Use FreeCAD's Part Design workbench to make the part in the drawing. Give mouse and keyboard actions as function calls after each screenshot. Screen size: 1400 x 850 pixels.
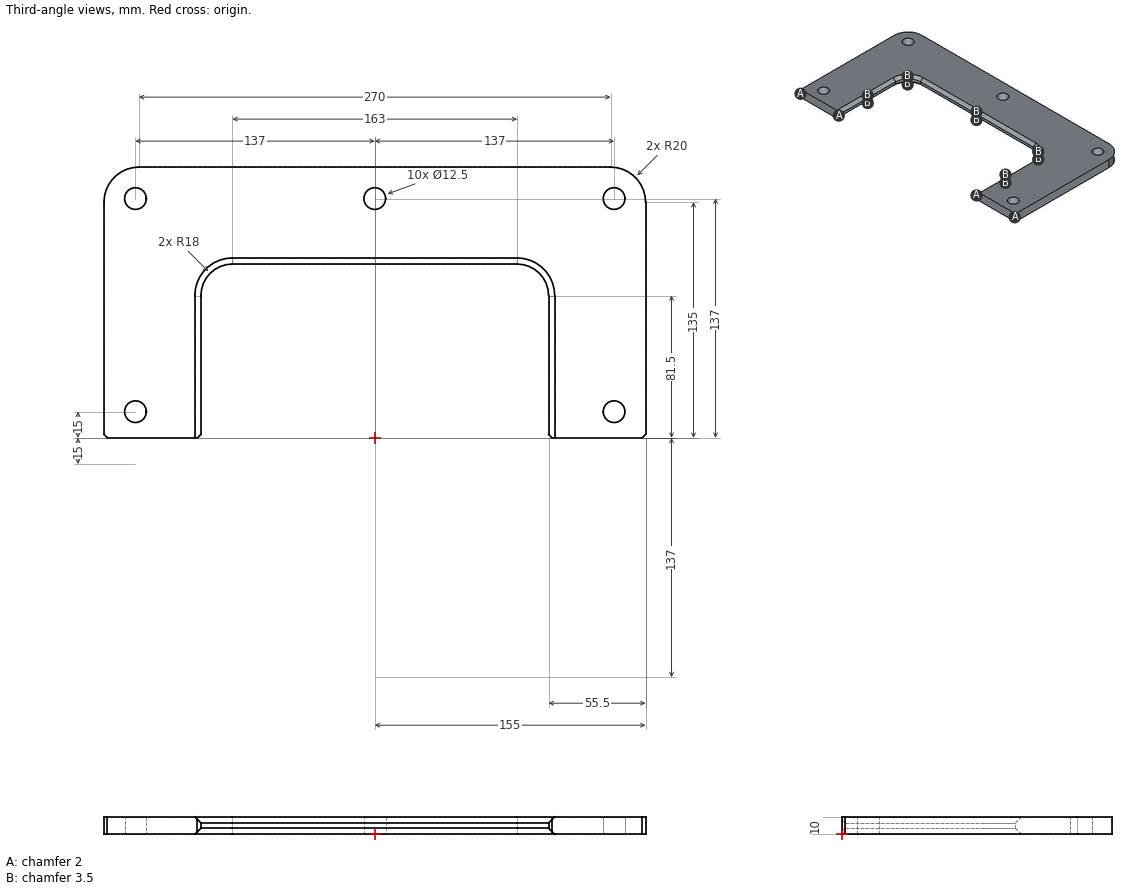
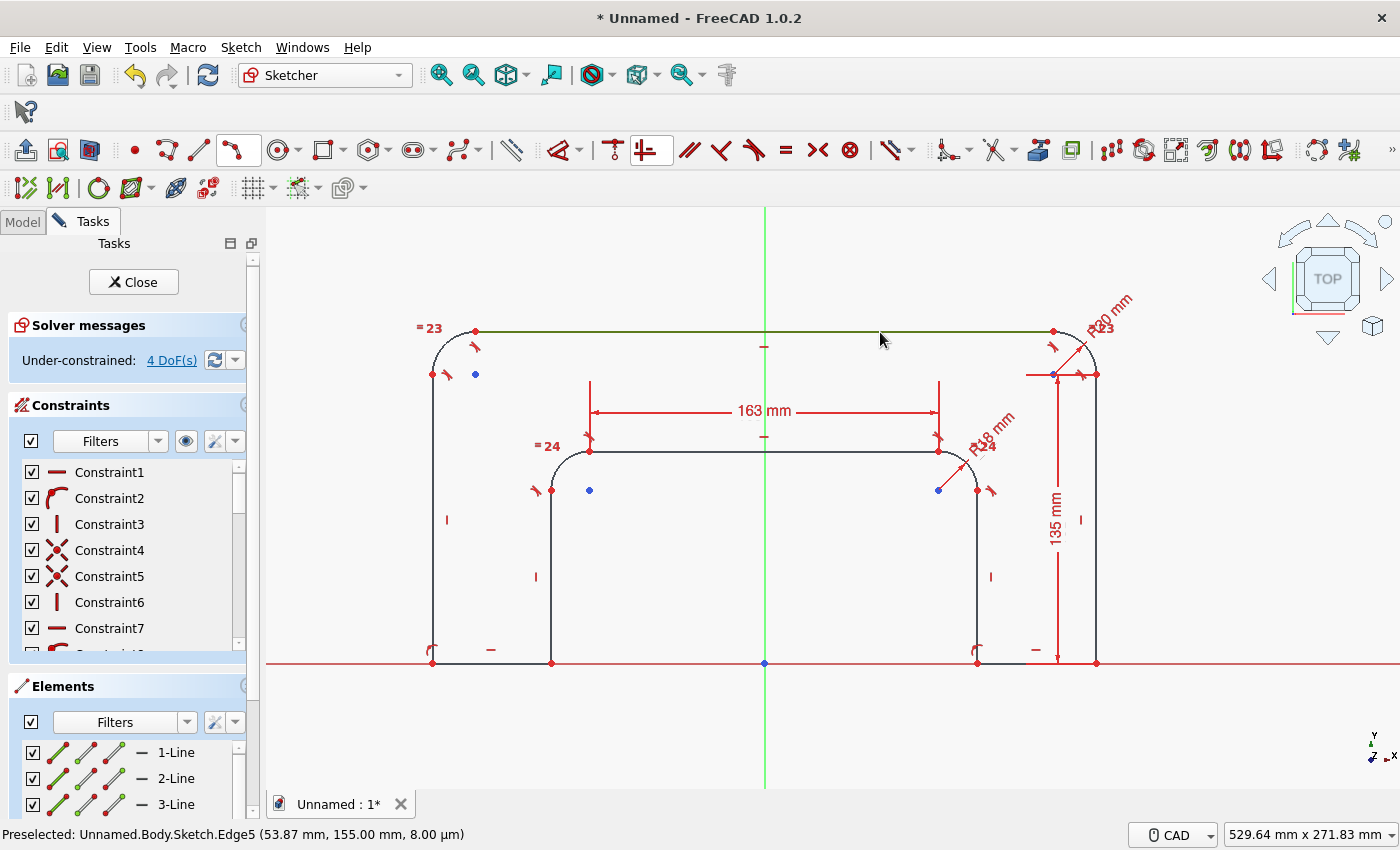
key(l)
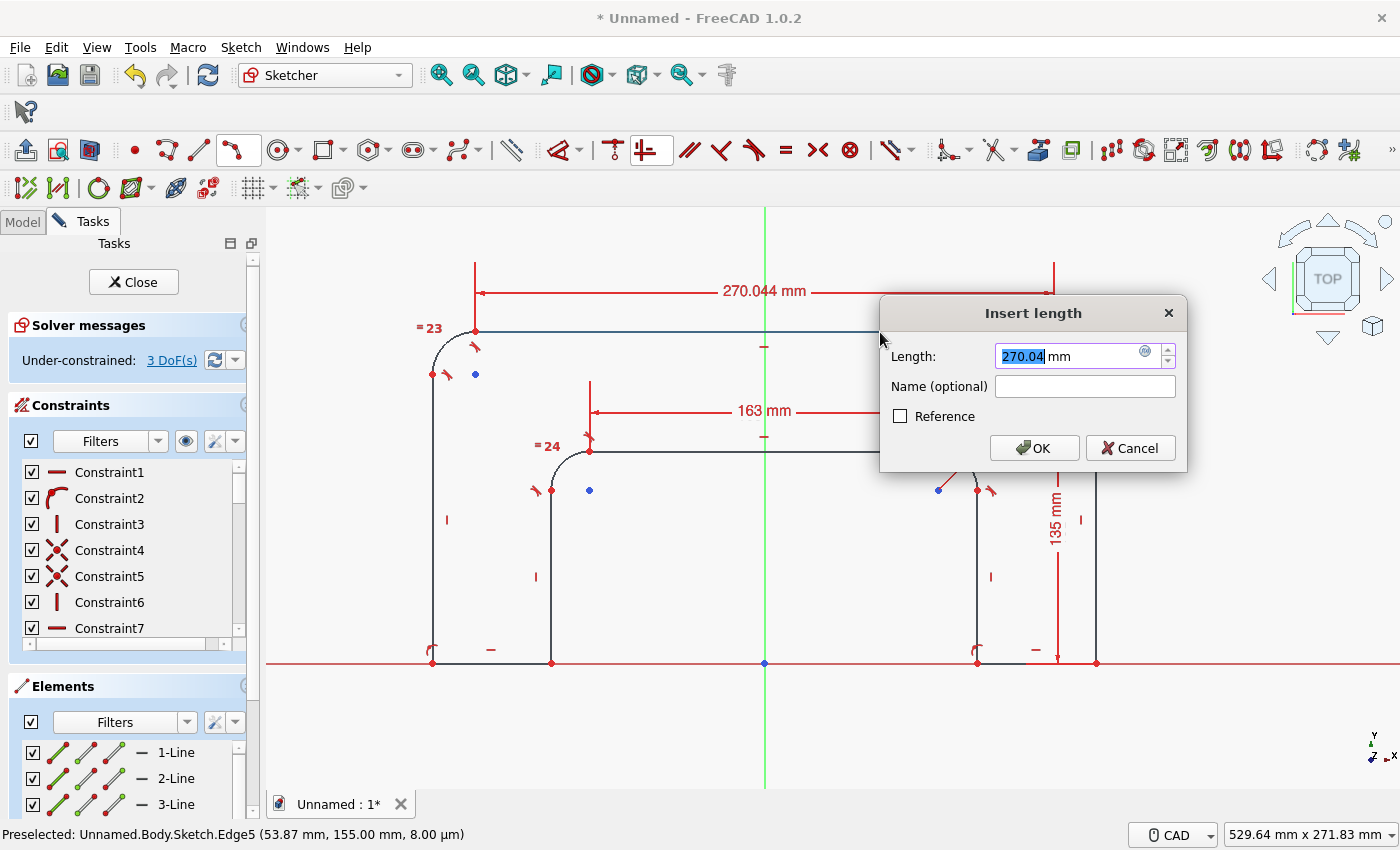
text(270)
key(Return)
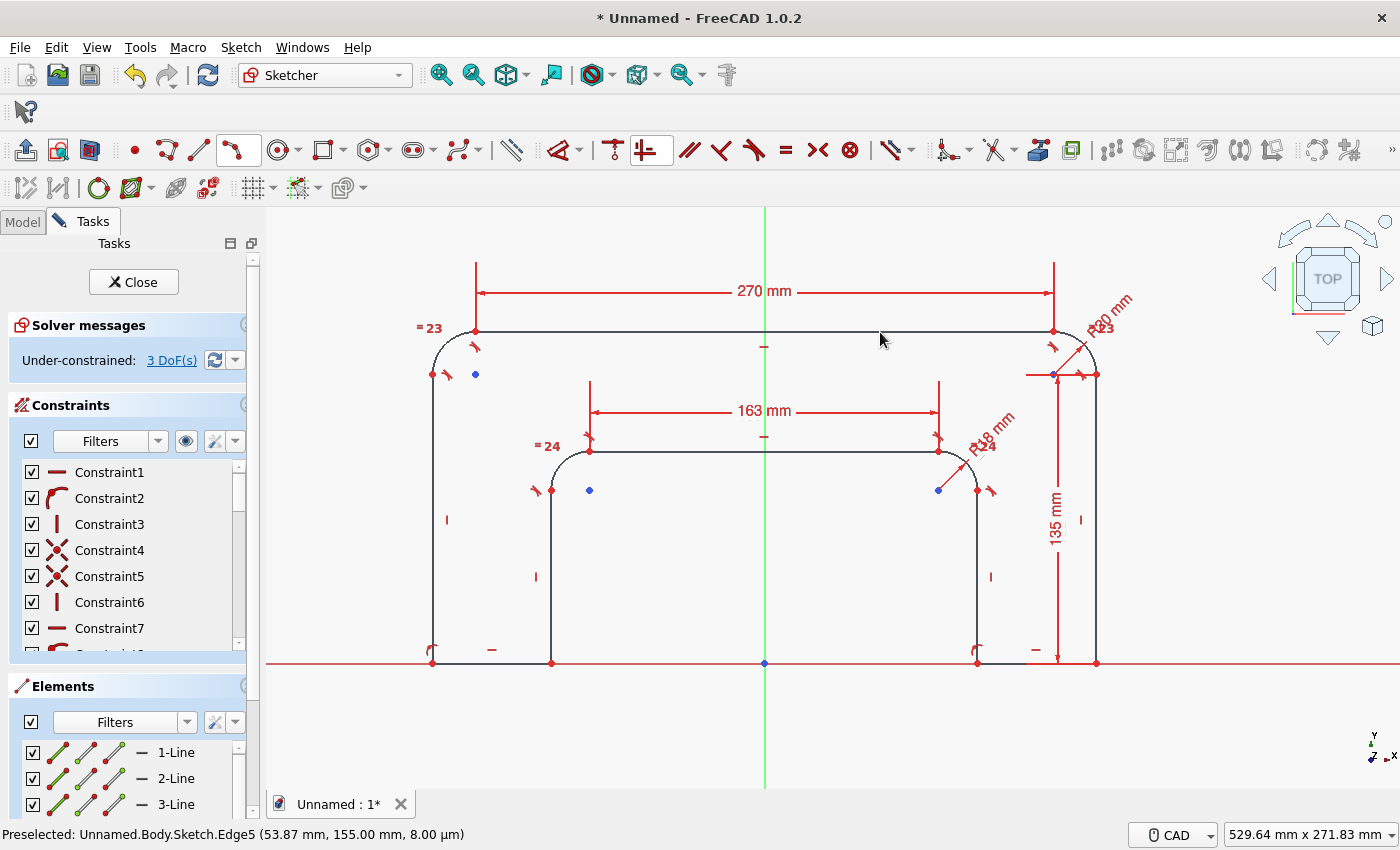
click(977, 542)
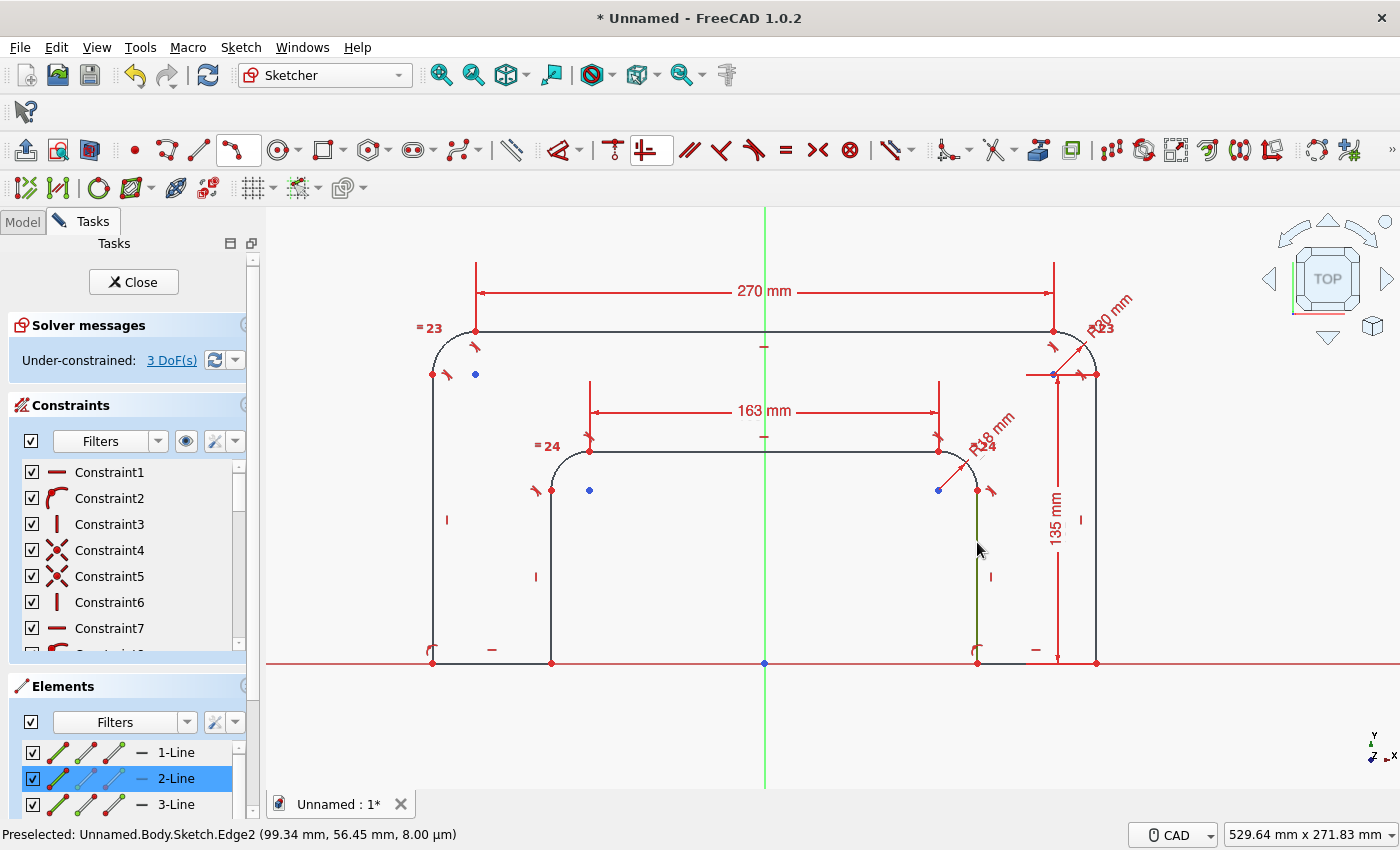
key(i)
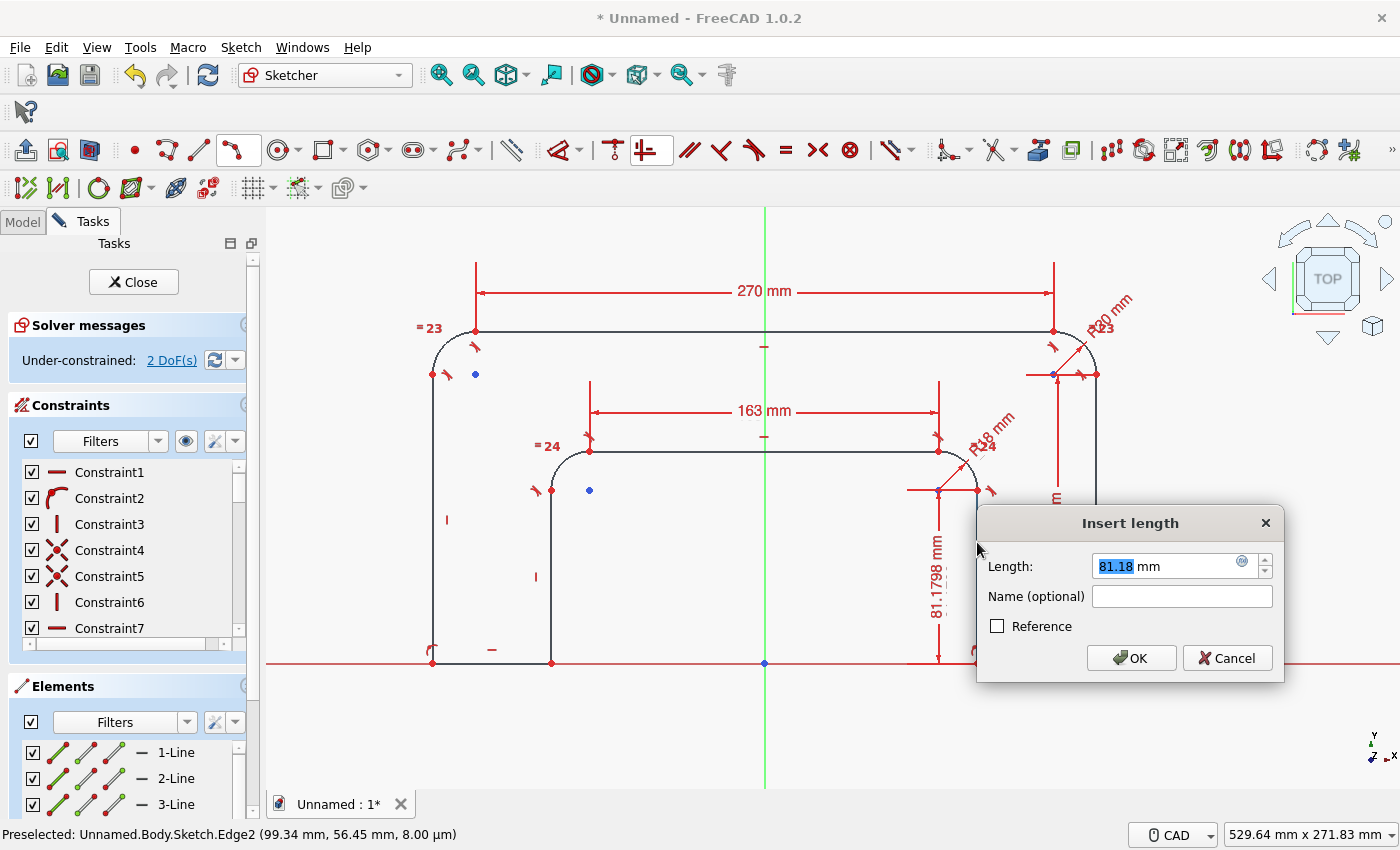
text(81.5)
key(Return)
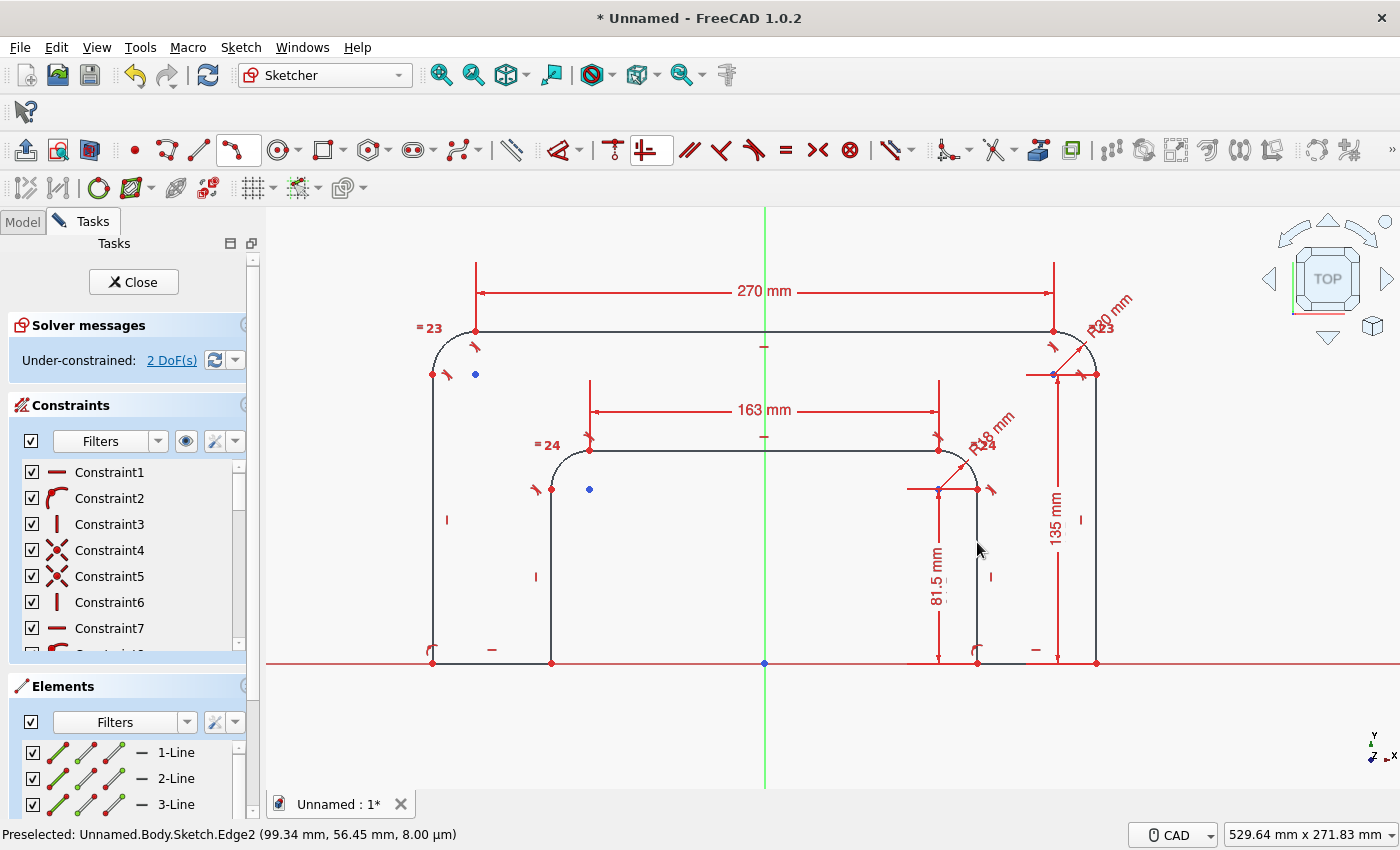
click(1013, 664)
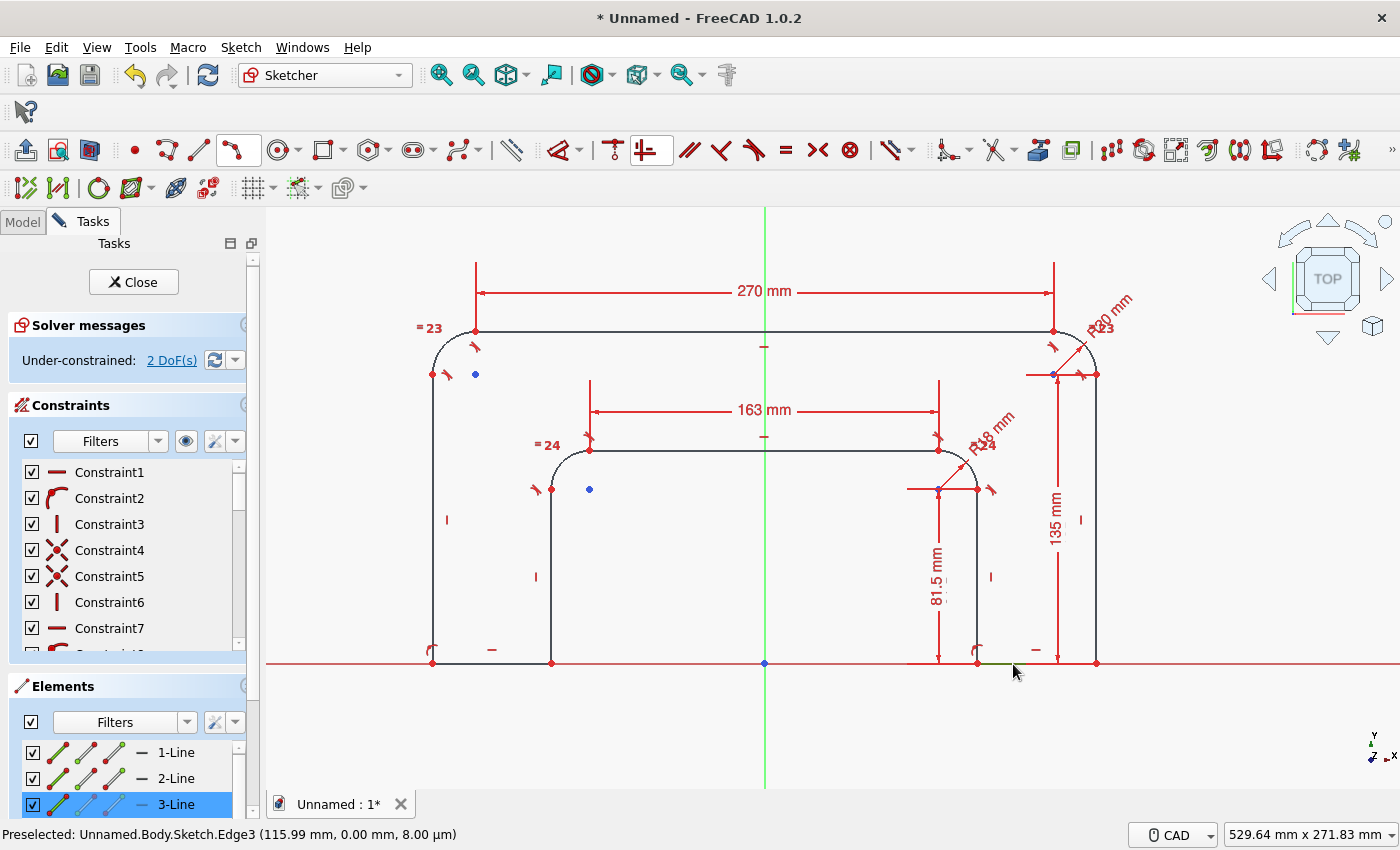
key(l)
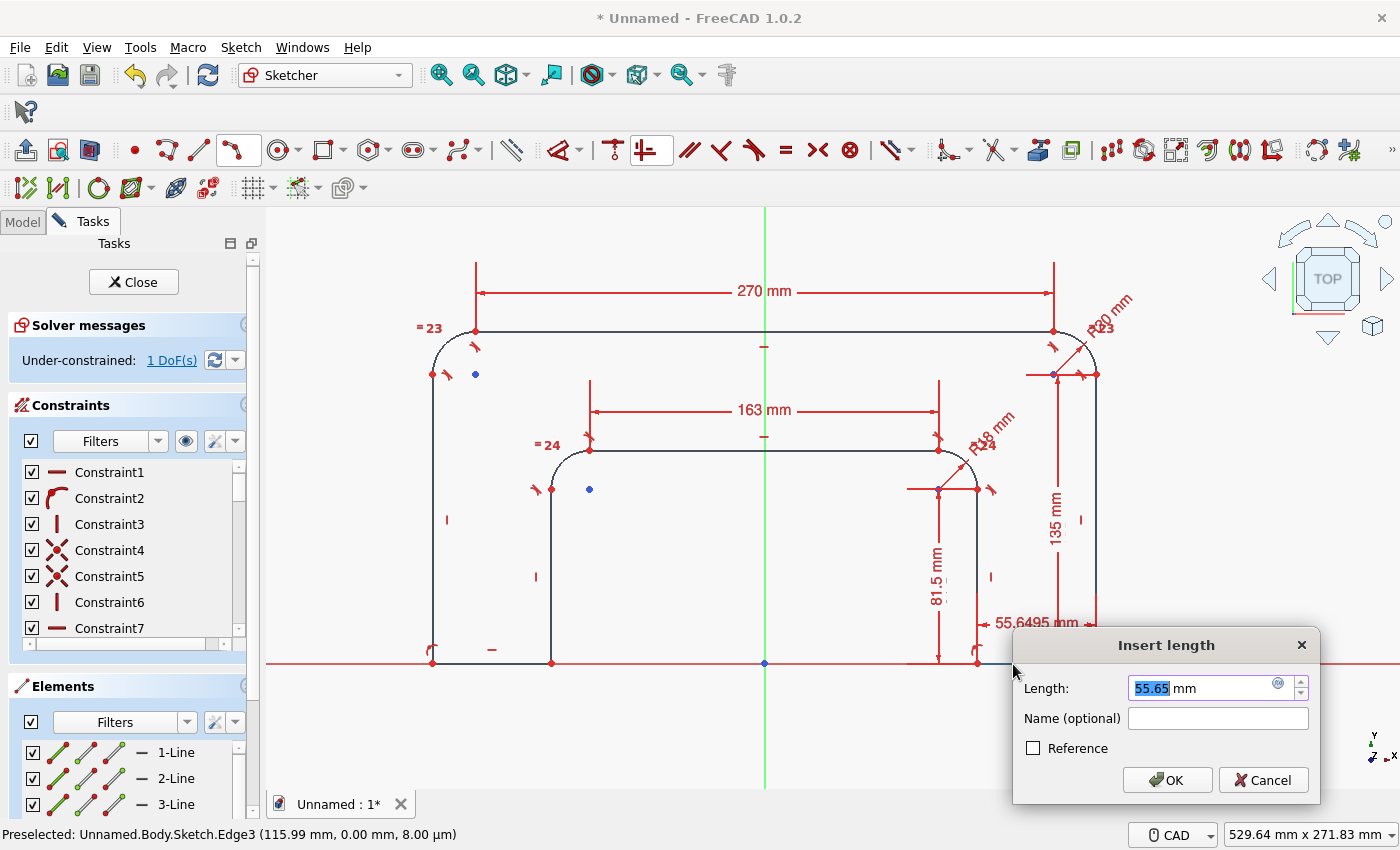
text(55.5)
key(Return)